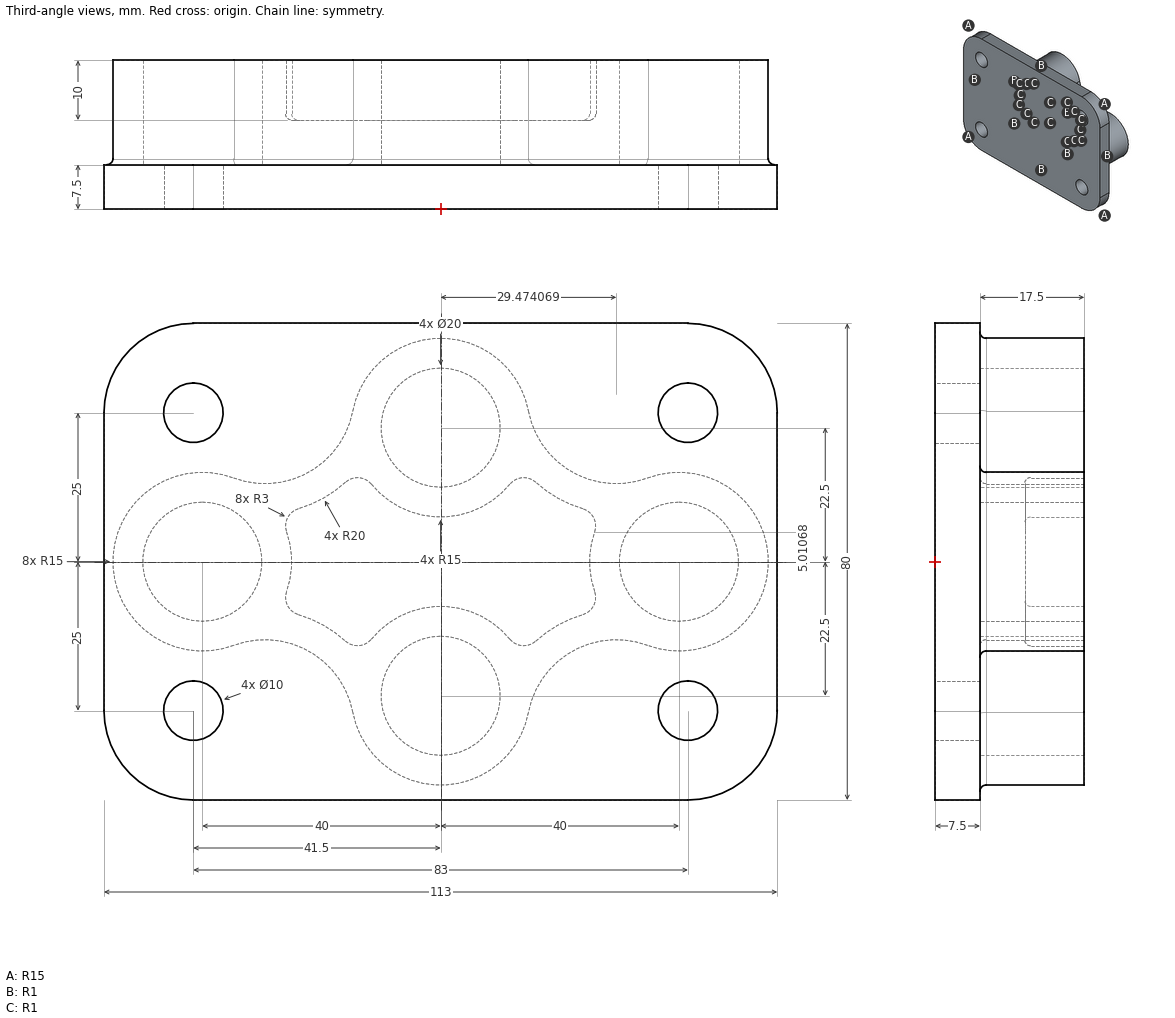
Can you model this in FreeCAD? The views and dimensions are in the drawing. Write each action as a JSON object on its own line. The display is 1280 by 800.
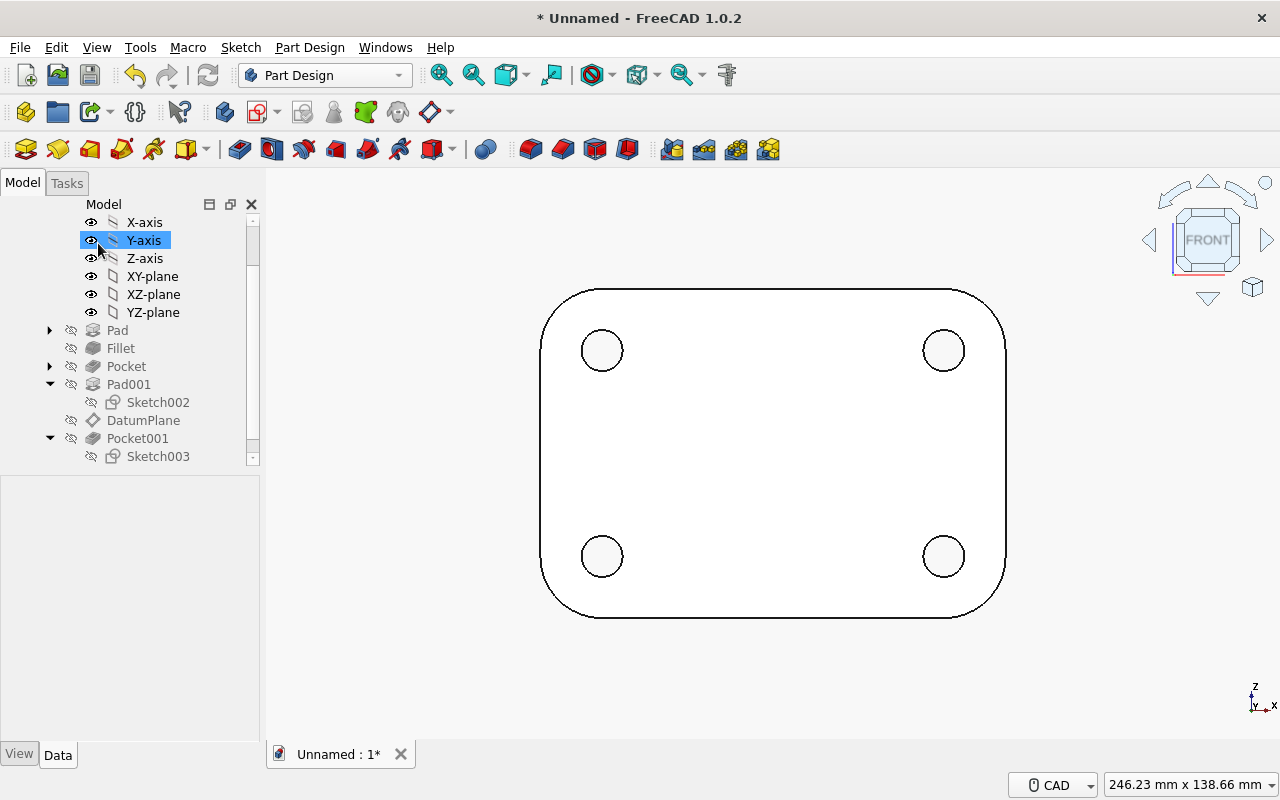
{"action": "key", "text": "3"}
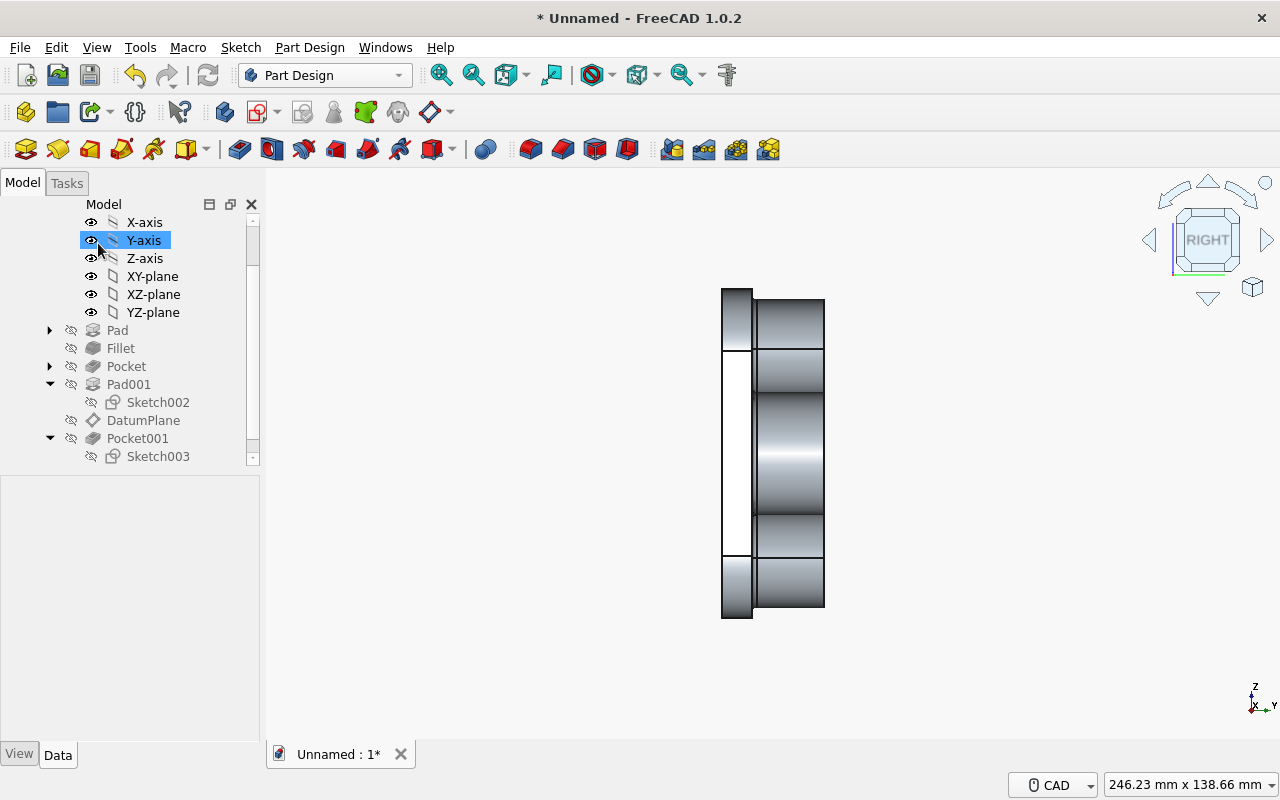
{"action": "key", "text": "5"}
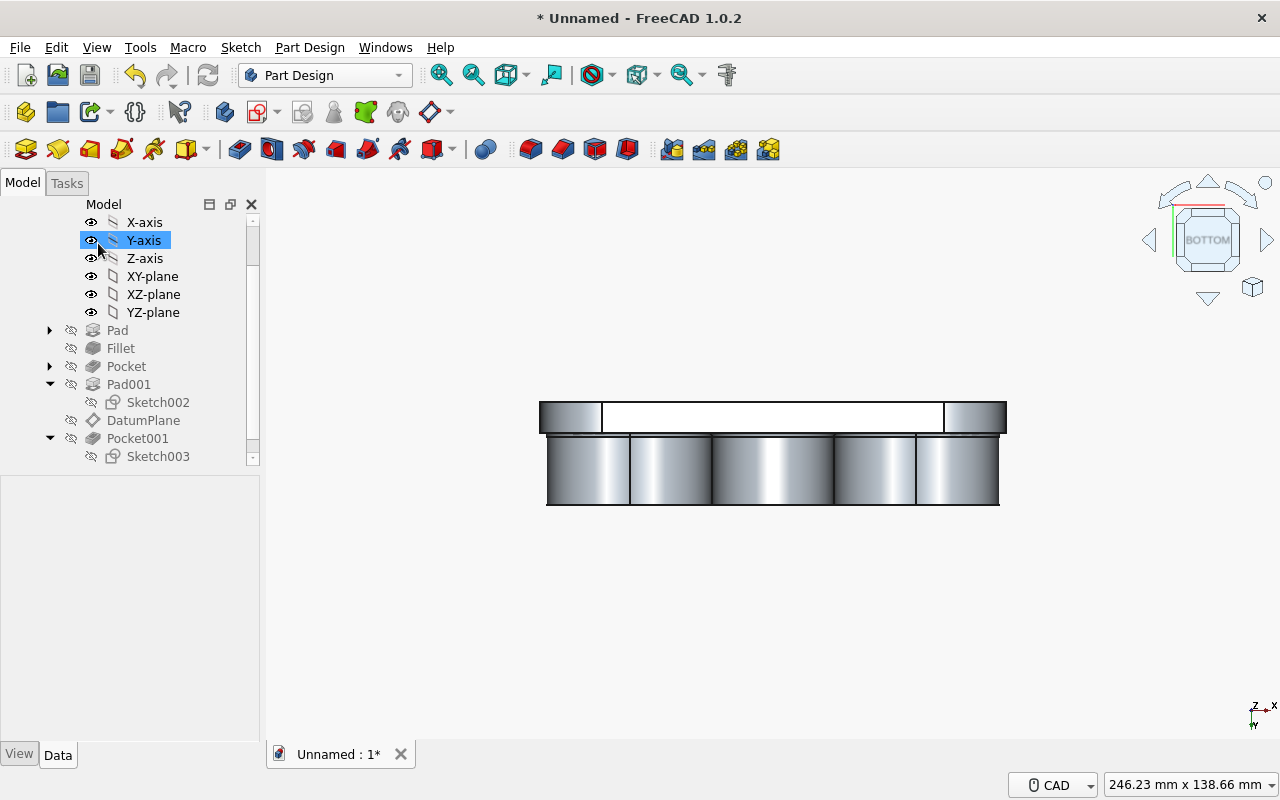
{"action": "key", "text": "4"}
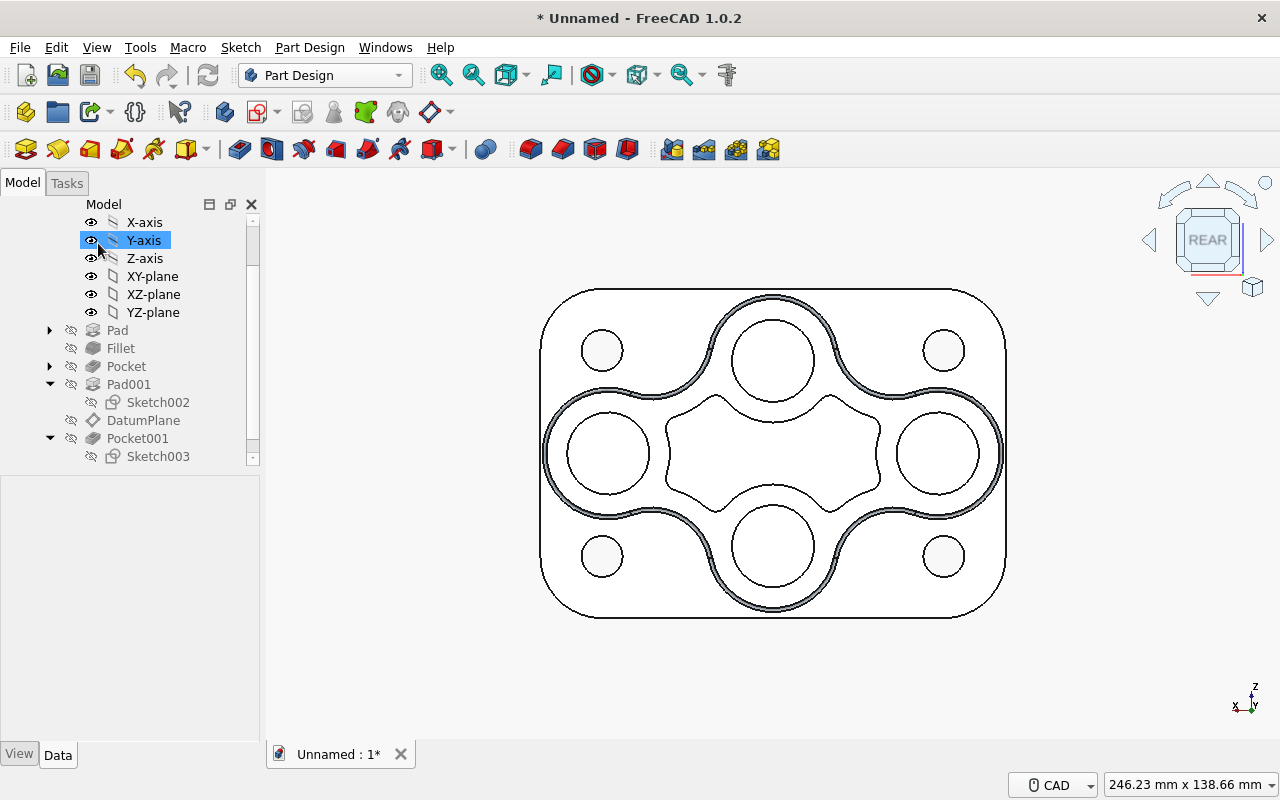
{"action": "left_click", "coordinate": [712, 452]}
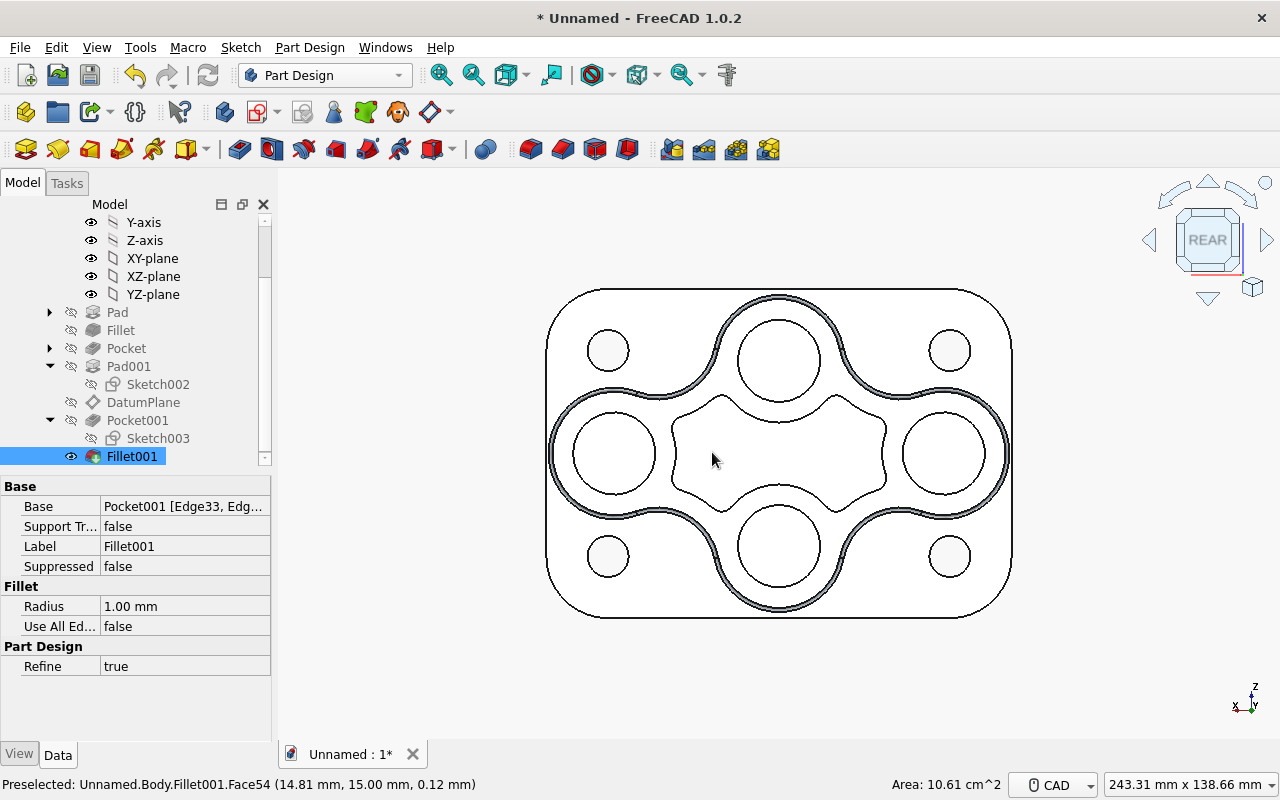
{"action": "left_click", "coordinate": [532, 150]}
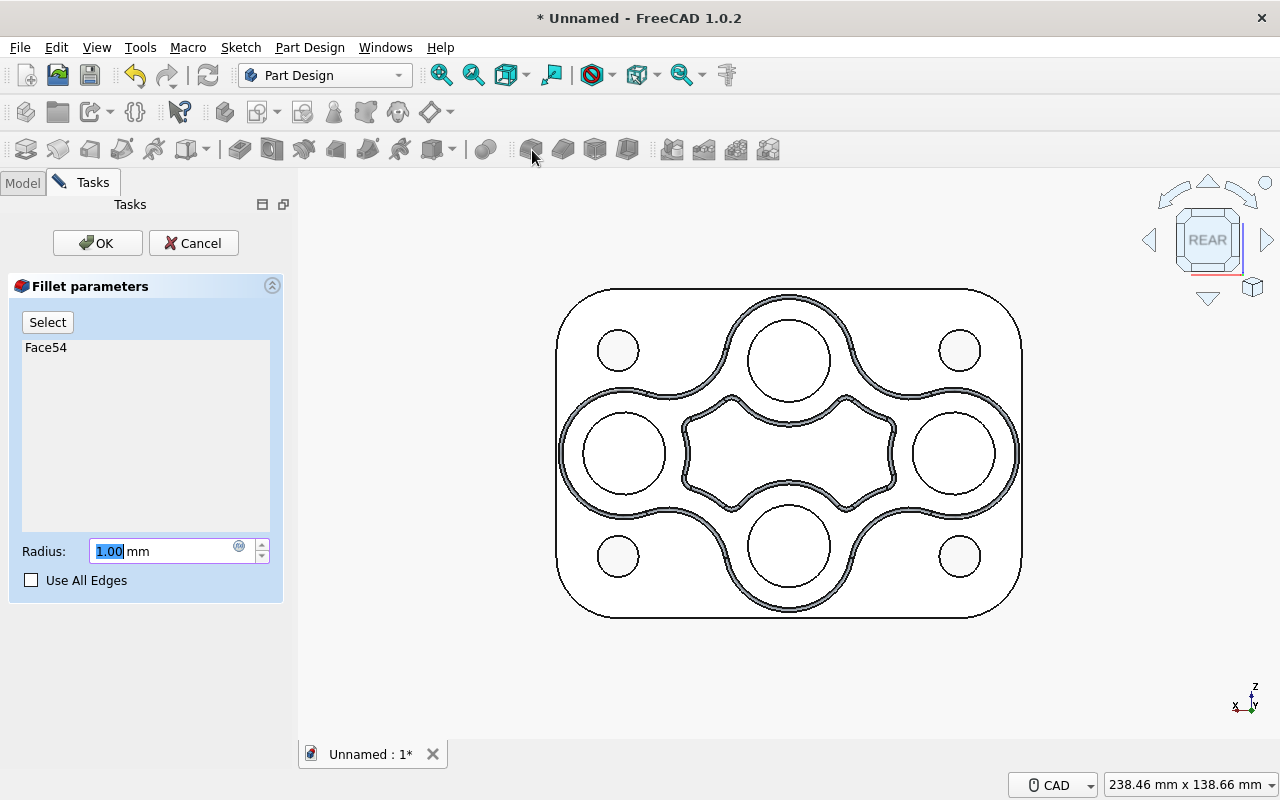
{"action": "type", "text": "1"}
{"action": "key", "text": "Tab"}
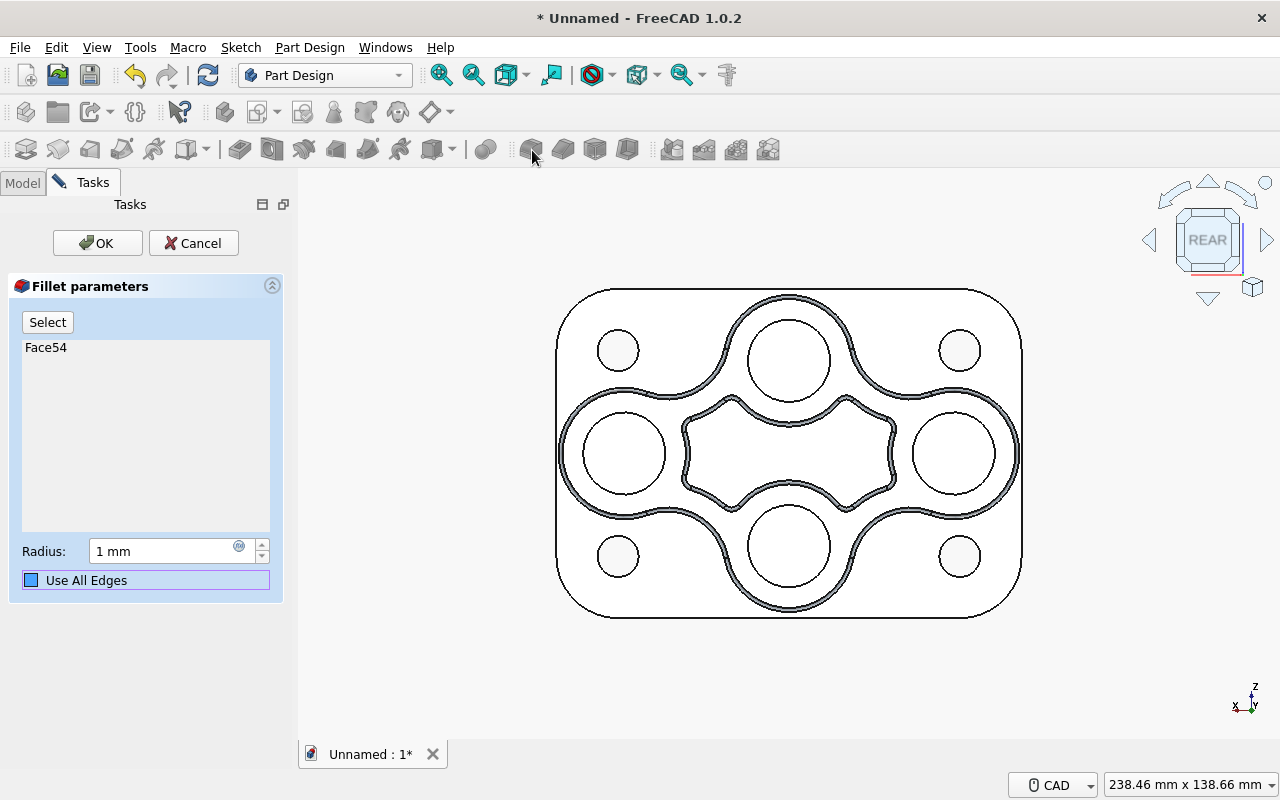
{"action": "left_click", "coordinate": [98, 243]}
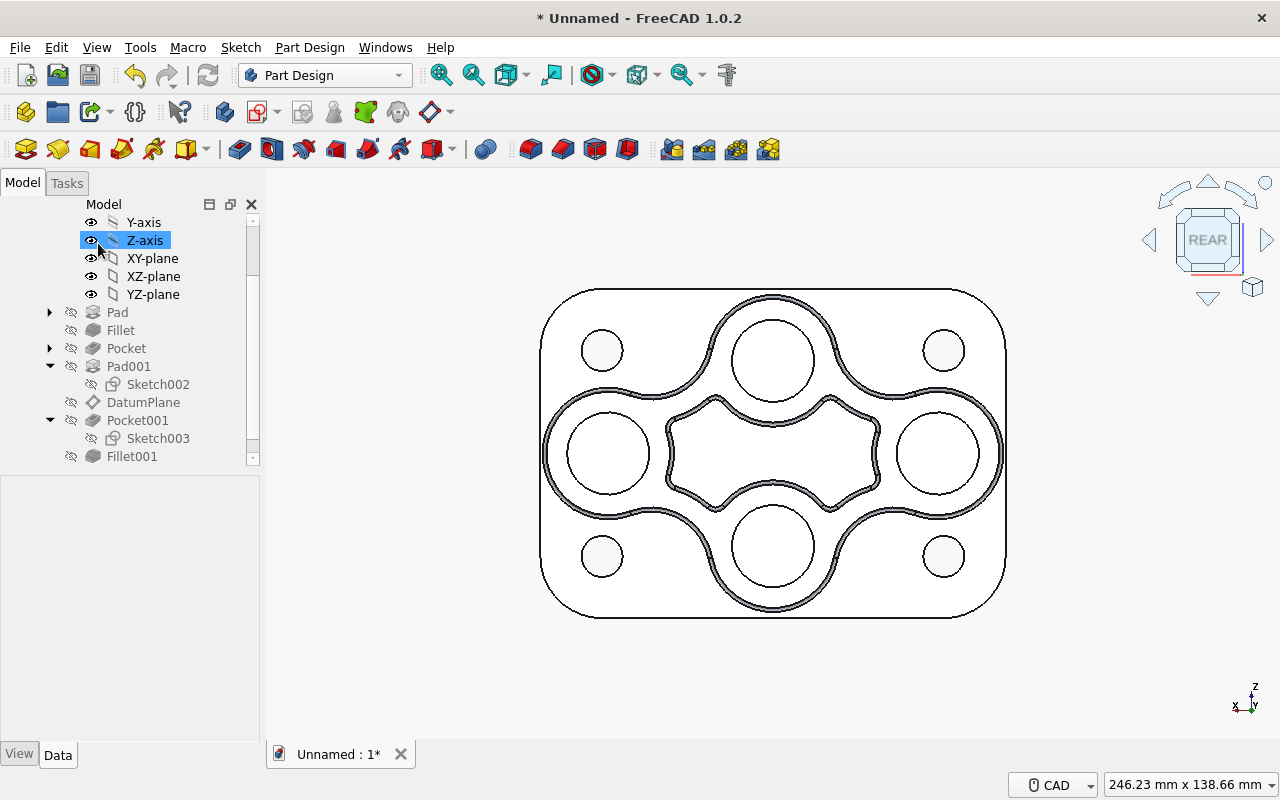
{"action": "key", "text": "0"}